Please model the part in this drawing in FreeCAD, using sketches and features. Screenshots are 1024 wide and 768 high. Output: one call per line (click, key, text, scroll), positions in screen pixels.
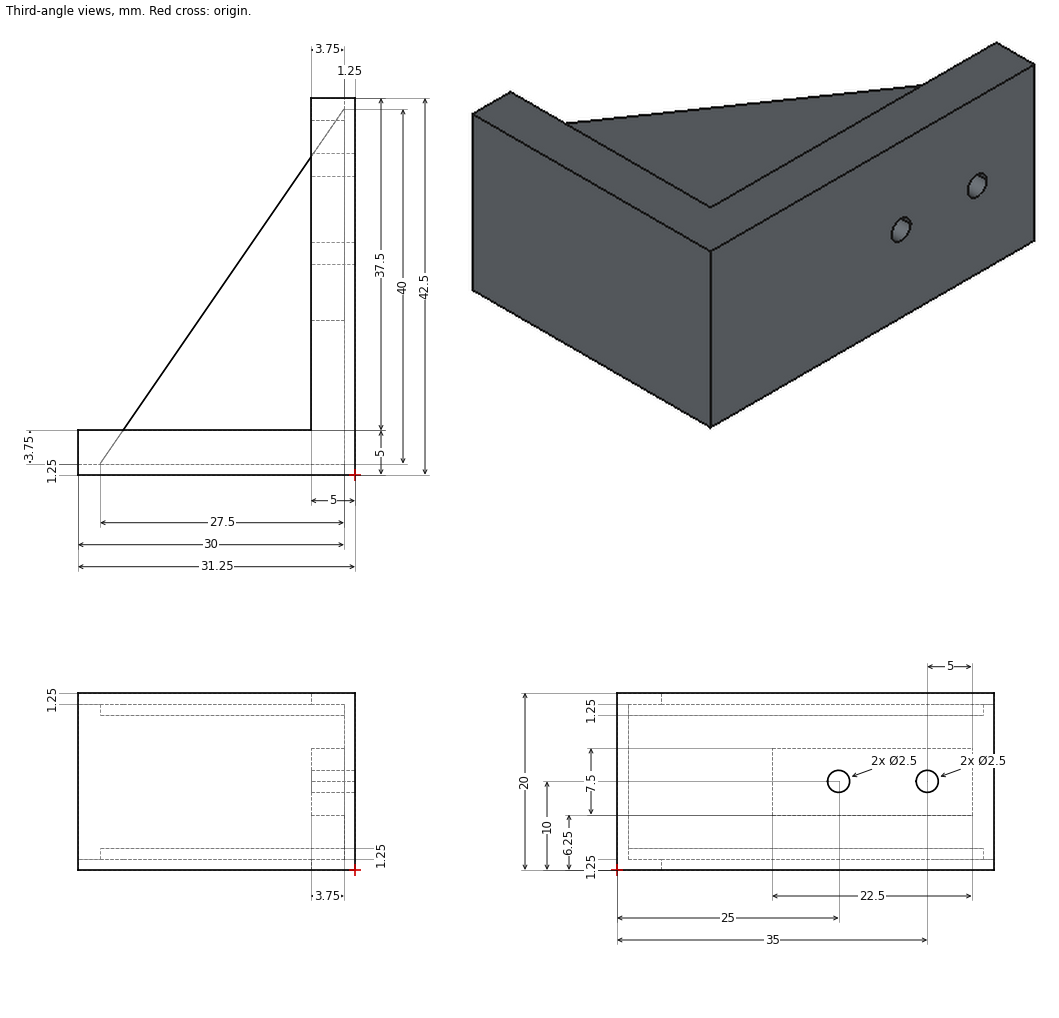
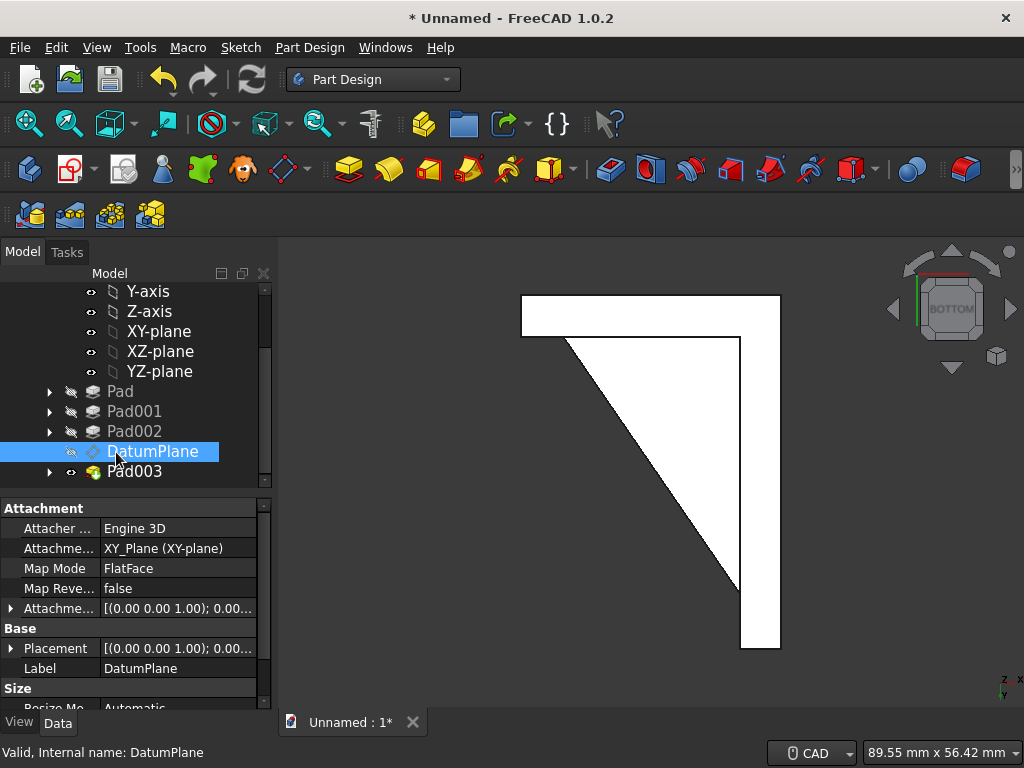
scroll(160, 387, down, 3)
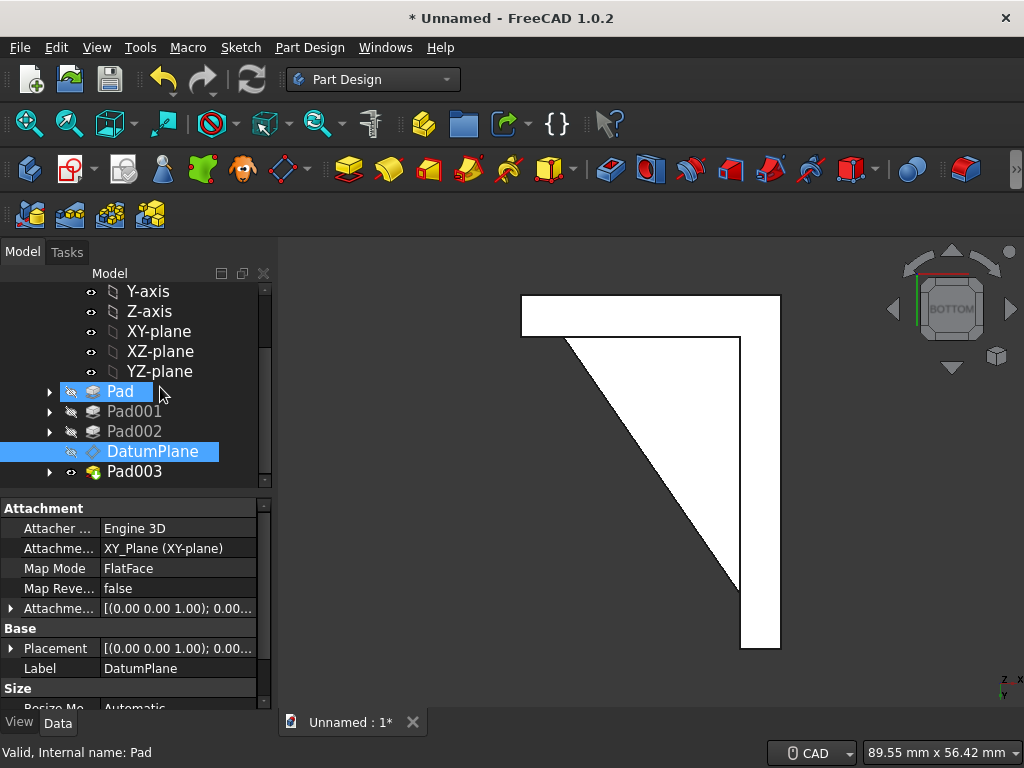
scroll(160, 387, up, 15)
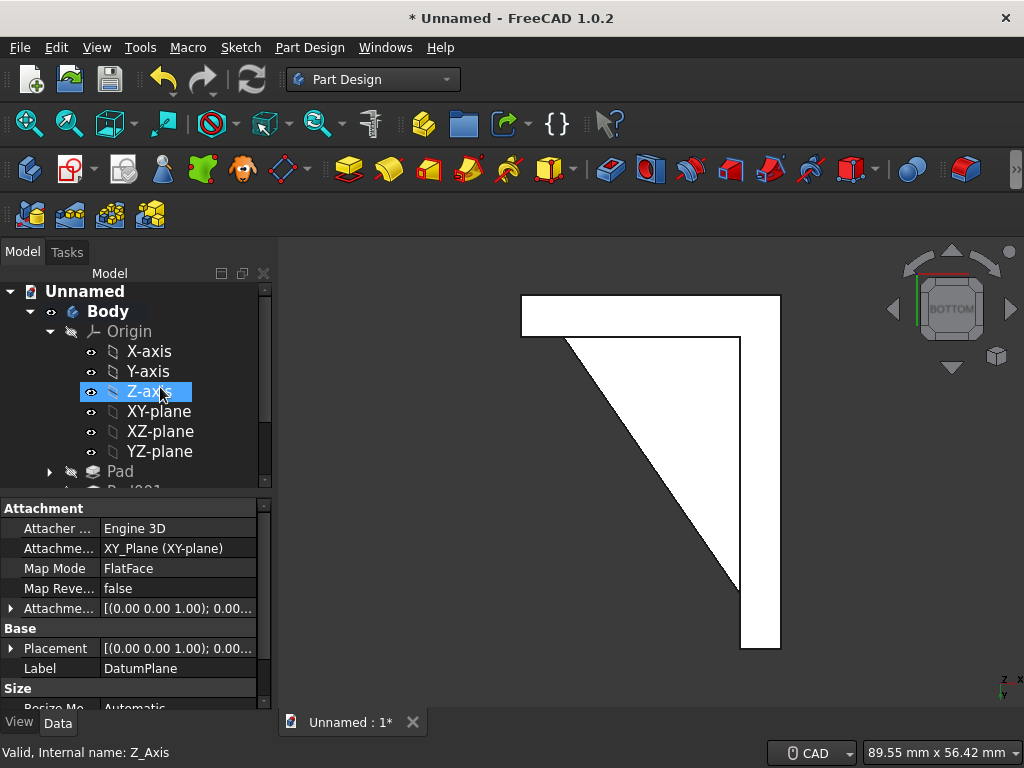
click(136, 412)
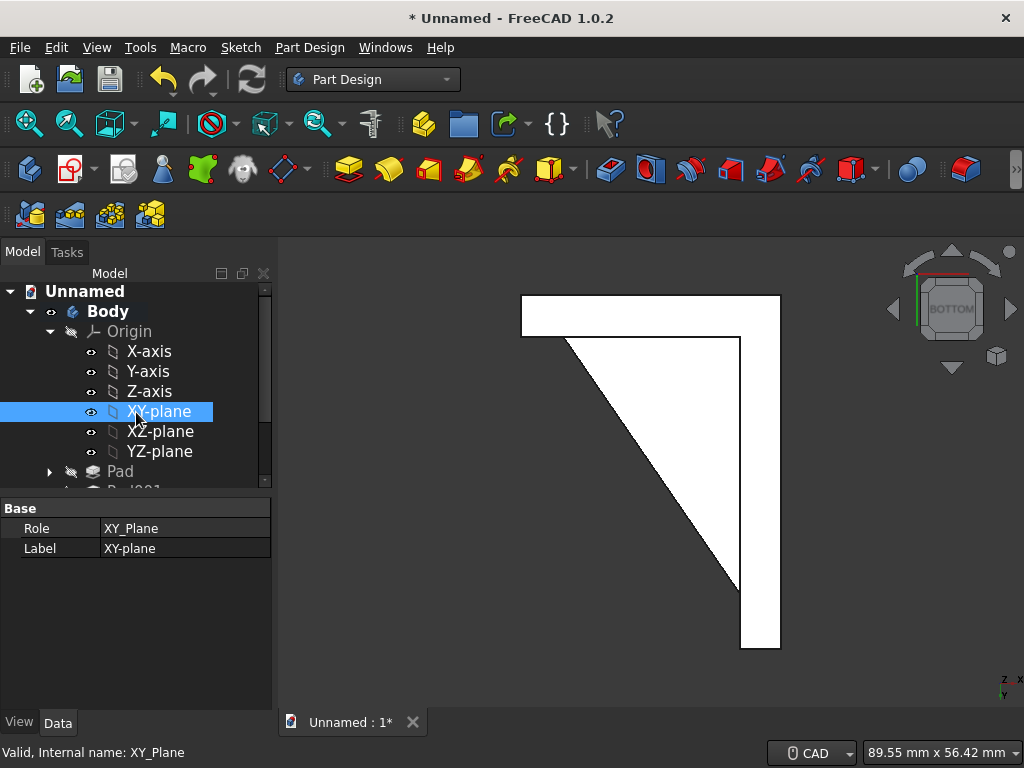
click(284, 170)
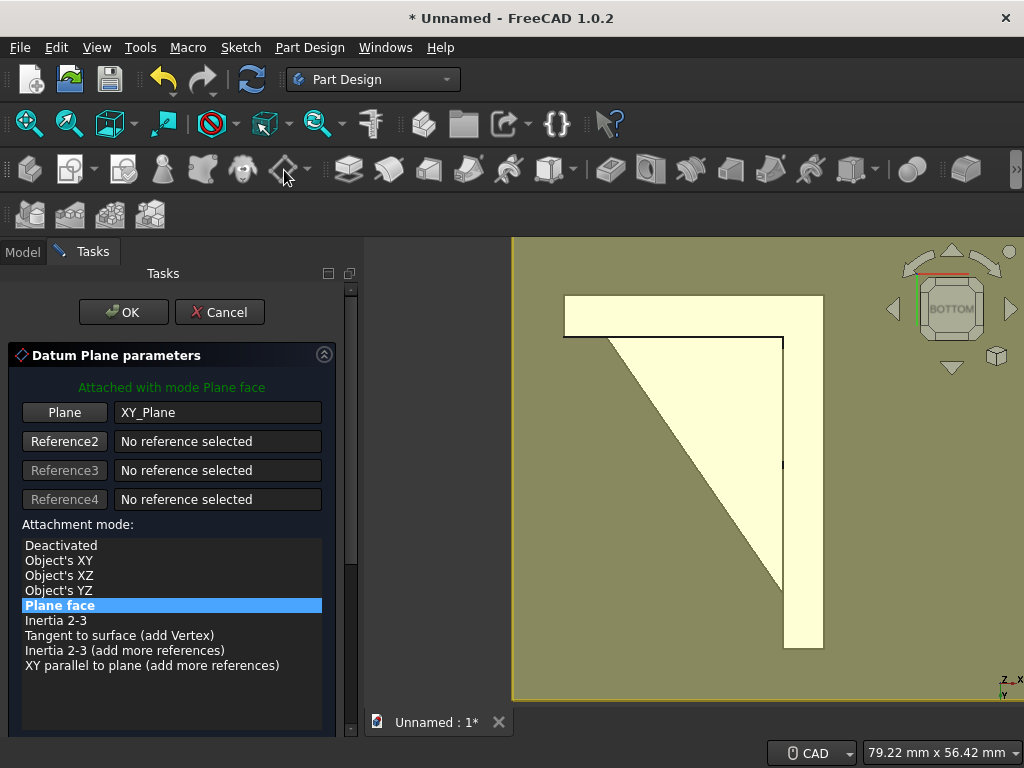
scroll(351, 510, down, 3)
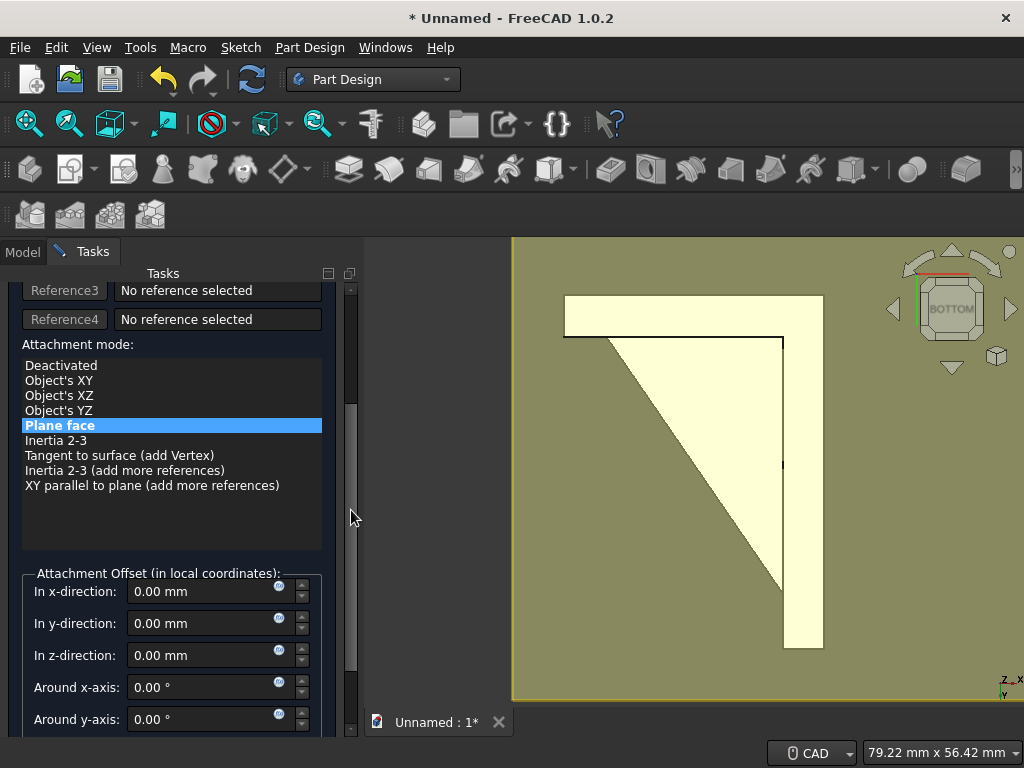
triple_click(210, 655)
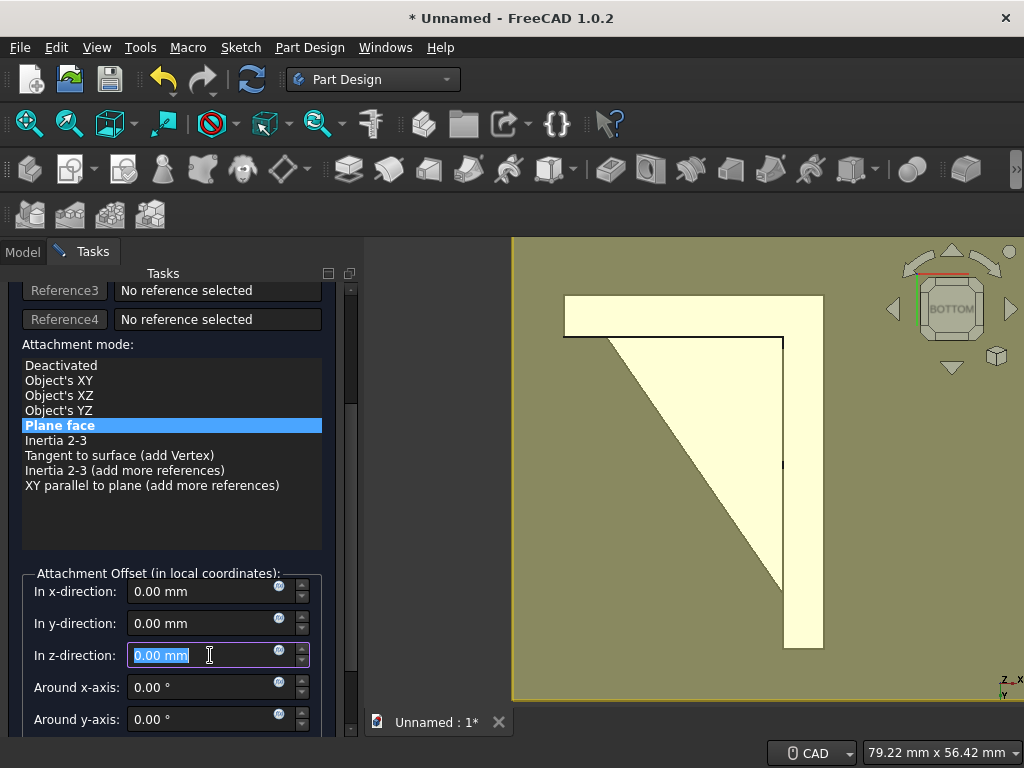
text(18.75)
key(Tab)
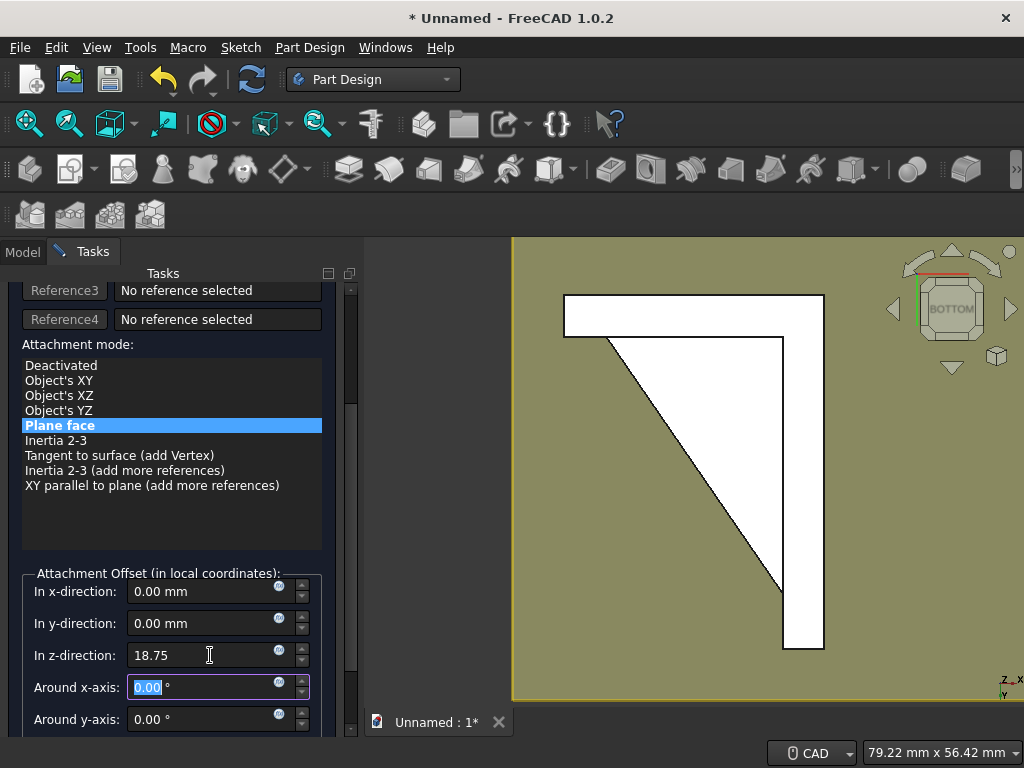
scroll(351, 510, up, 4)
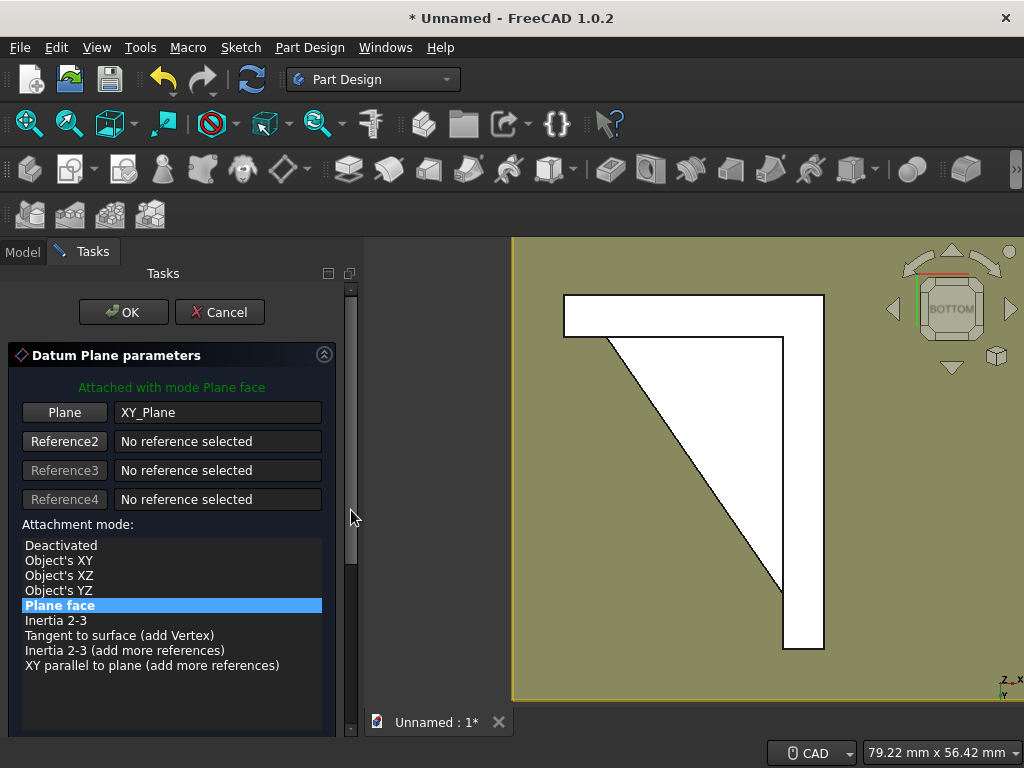
click(124, 312)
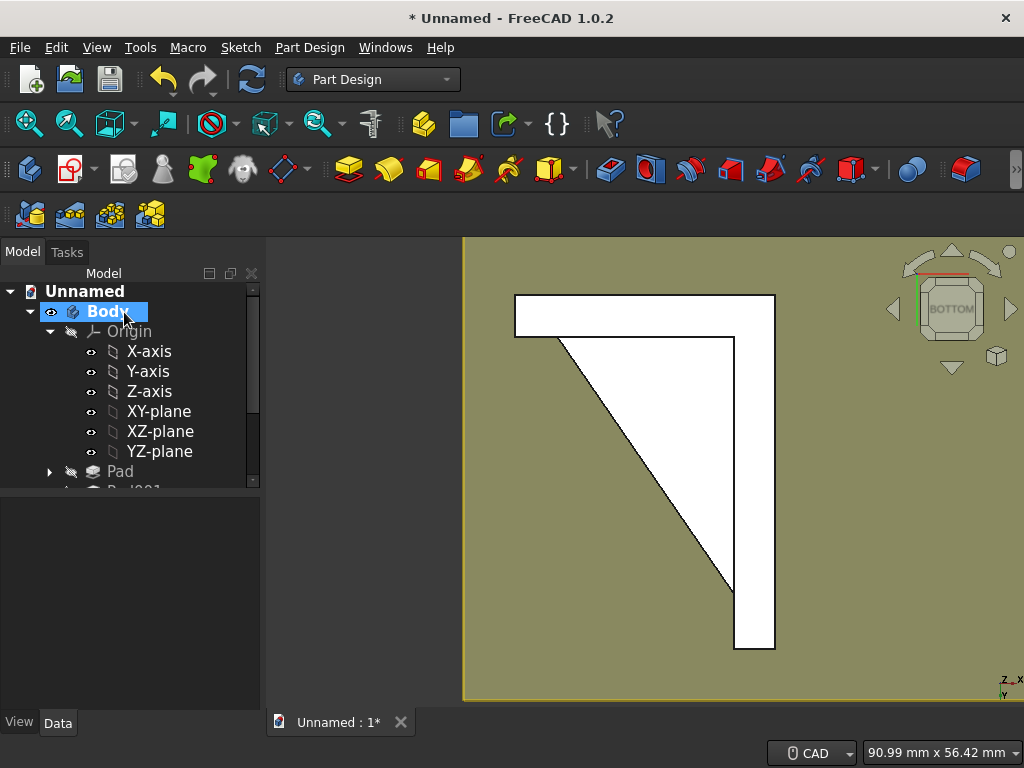
scroll(100, 387, down, 3)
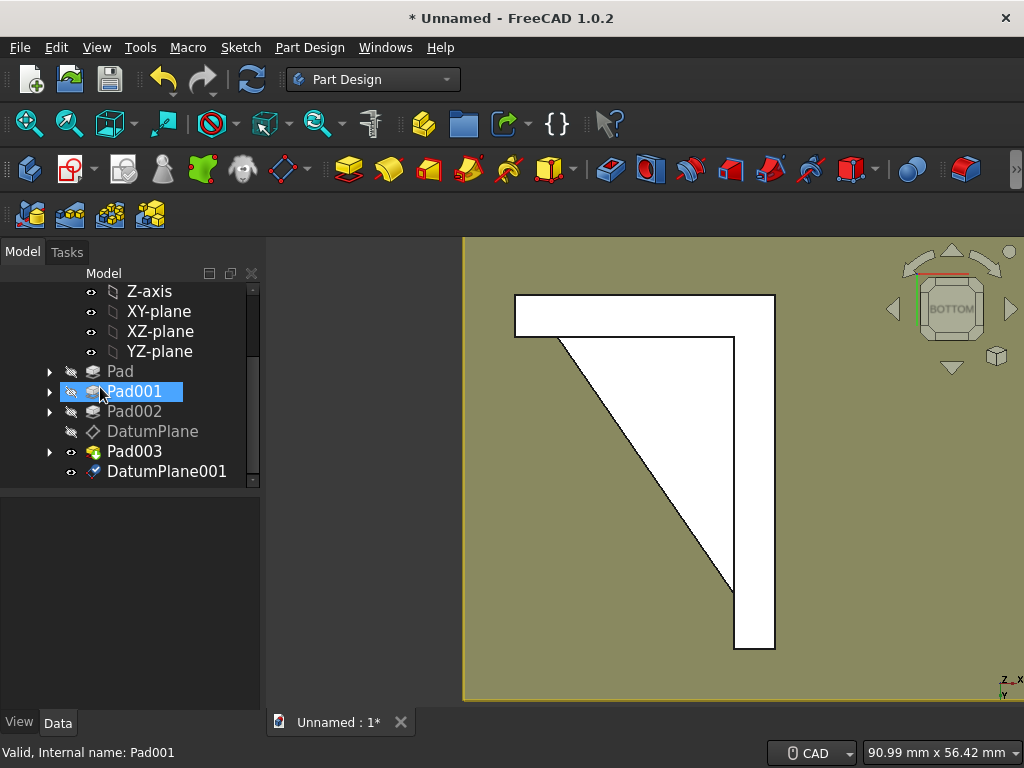
click(116, 472)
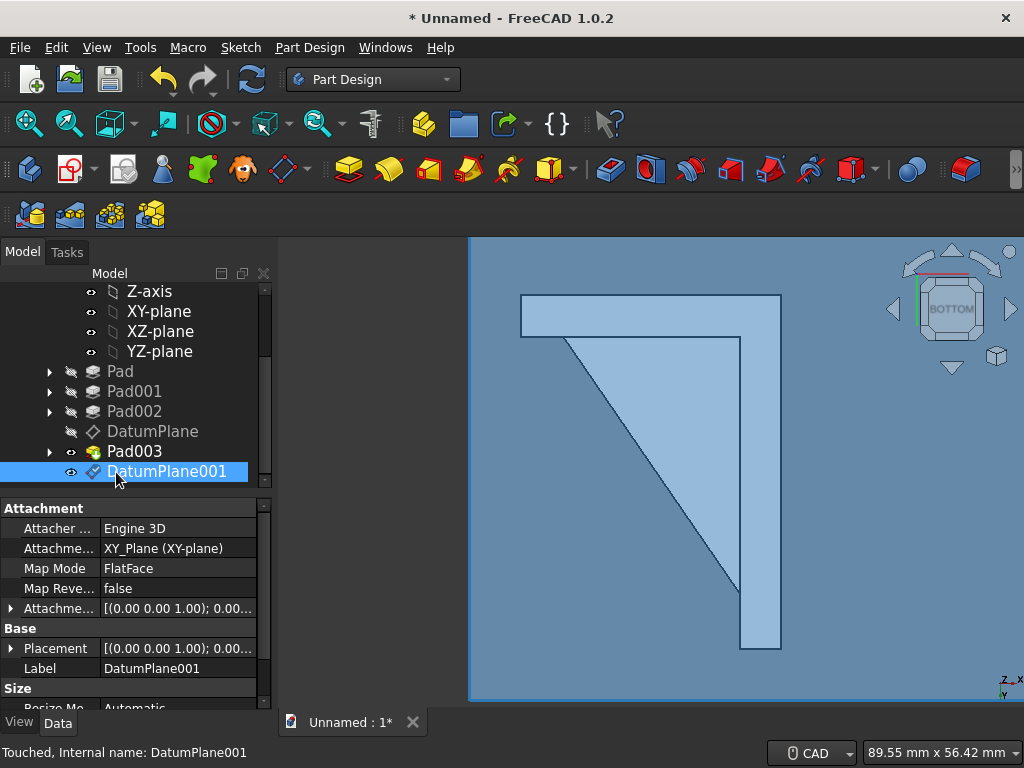
click(70, 170)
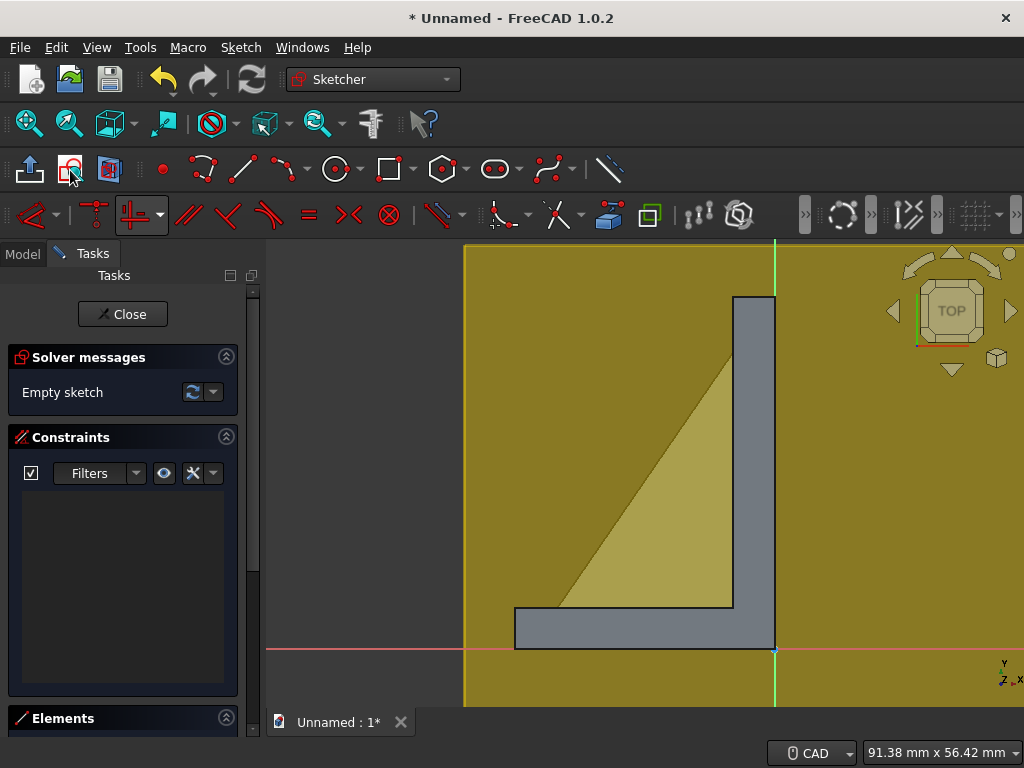
click(110, 170)